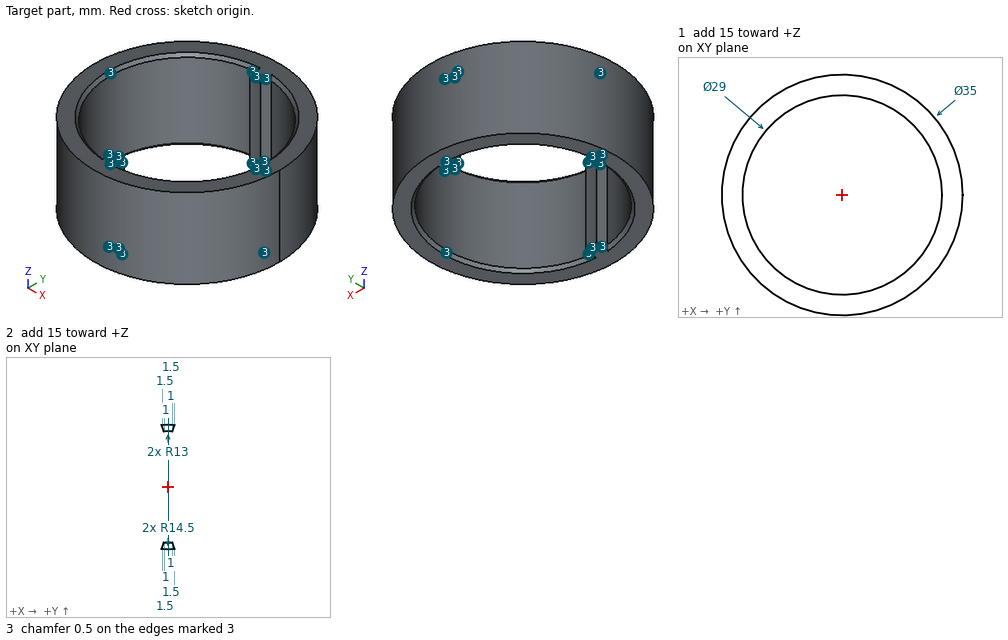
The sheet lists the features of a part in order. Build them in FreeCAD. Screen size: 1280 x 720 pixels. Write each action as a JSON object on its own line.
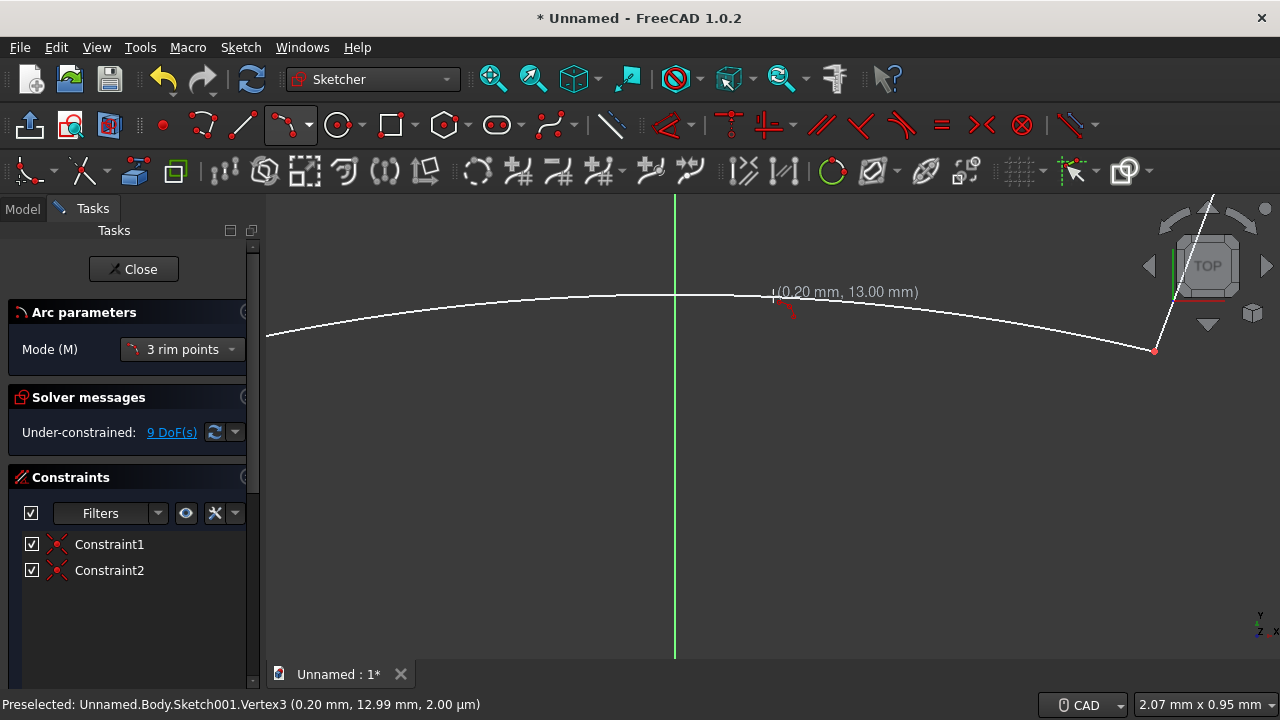
{"action": "scroll", "coordinate": [704, 426], "scroll_direction": "down", "scroll_amount": 15}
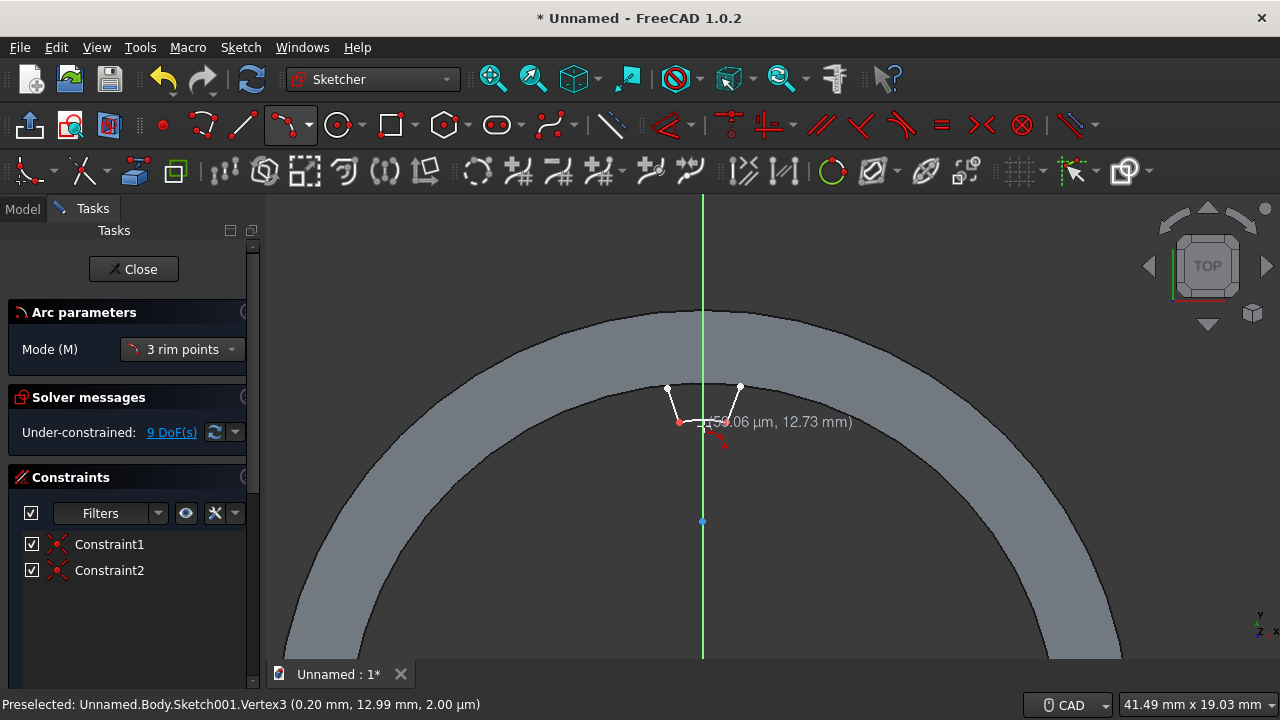
{"action": "scroll", "coordinate": [705, 245], "scroll_direction": "down", "scroll_amount": 5}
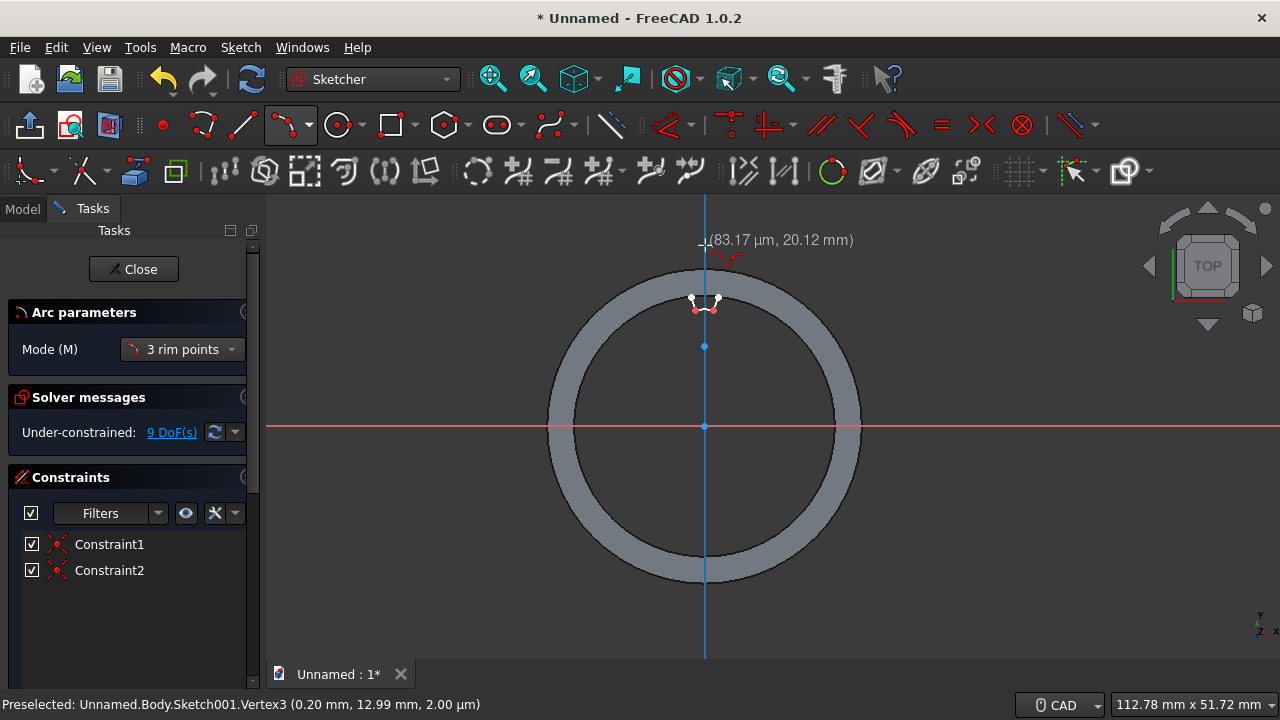
{"action": "scroll", "coordinate": [718, 297], "scroll_direction": "up", "scroll_amount": 5}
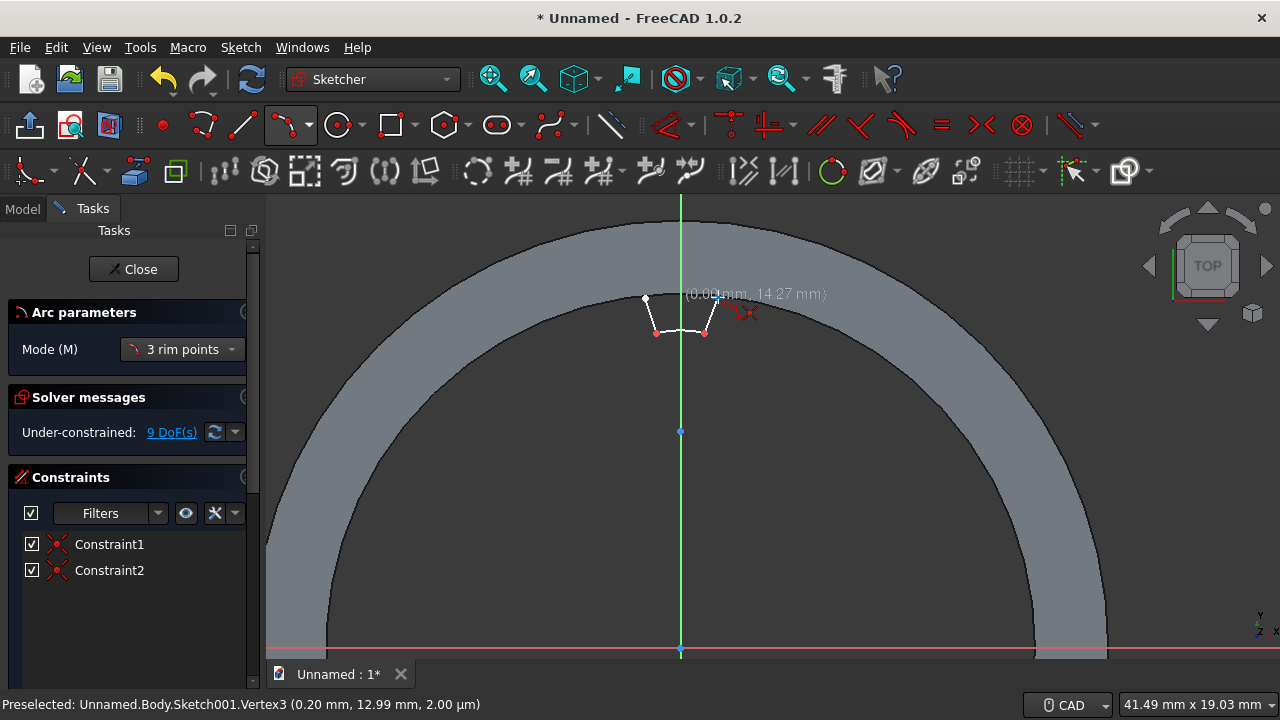
{"action": "left_click", "coordinate": [718, 297]}
{"action": "left_click", "coordinate": [645, 299]}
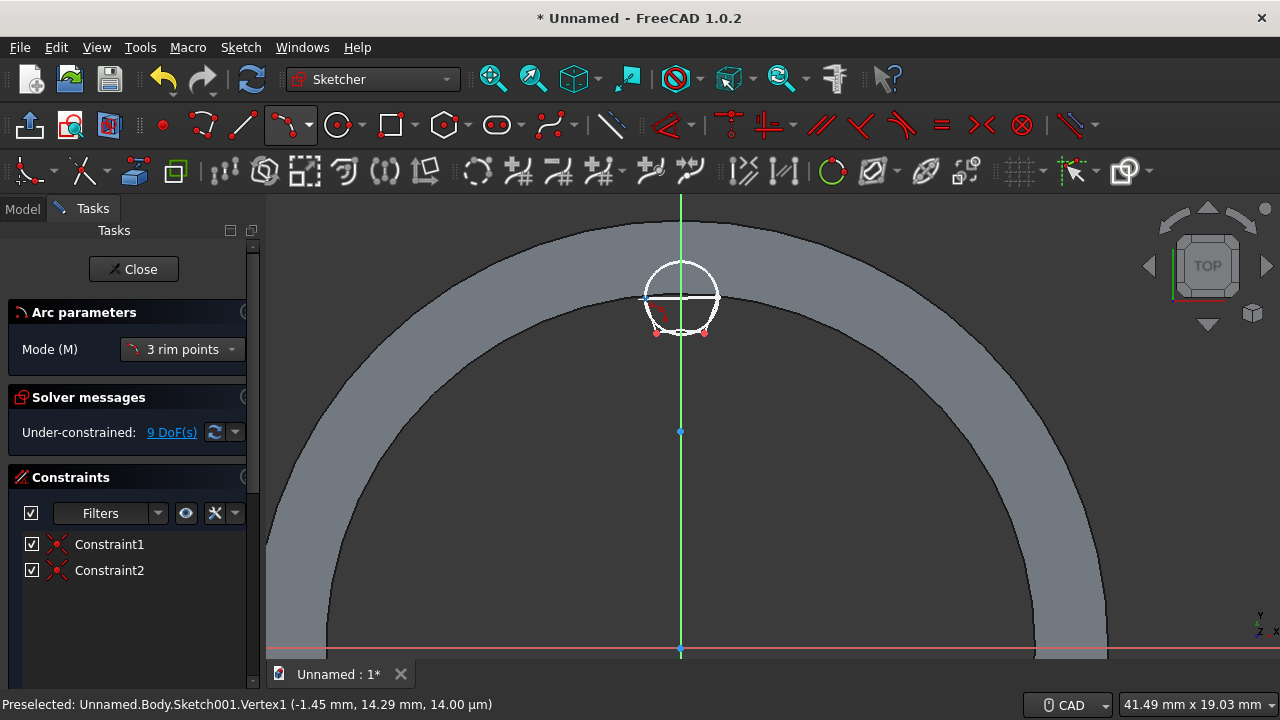
{"action": "scroll", "coordinate": [688, 294], "scroll_direction": "up", "scroll_amount": 11}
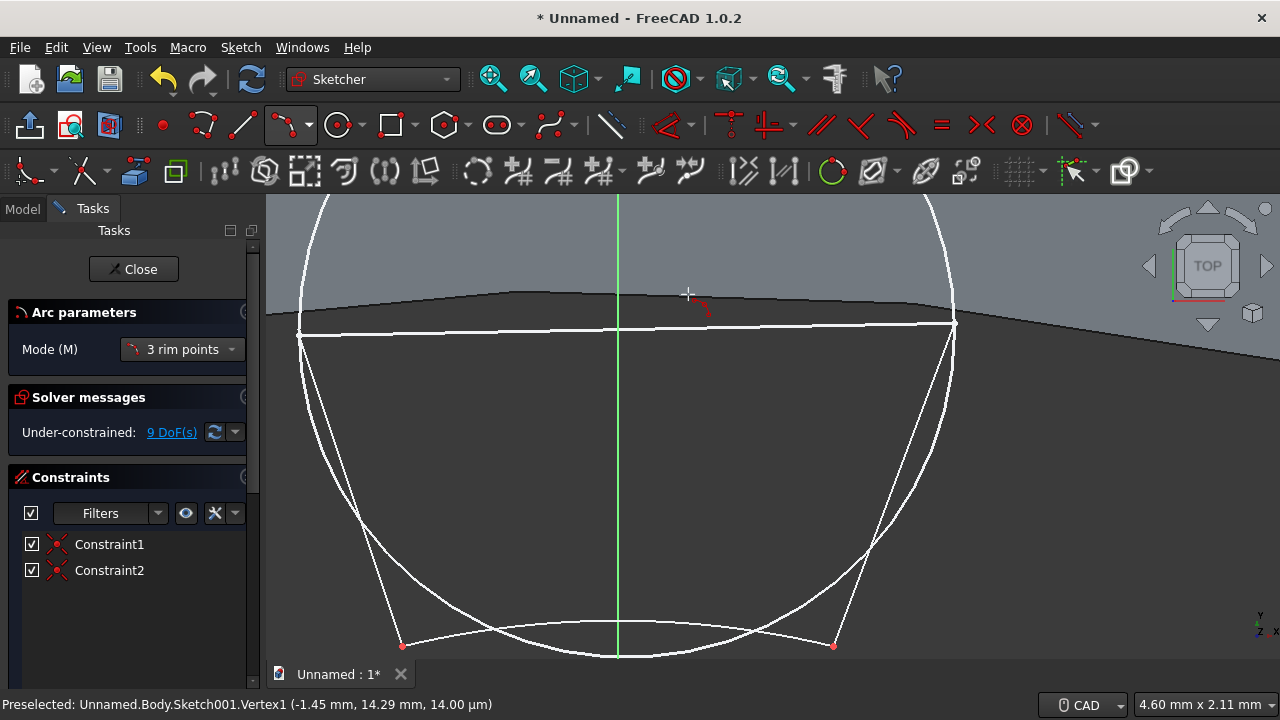
{"action": "left_click", "coordinate": [684, 291]}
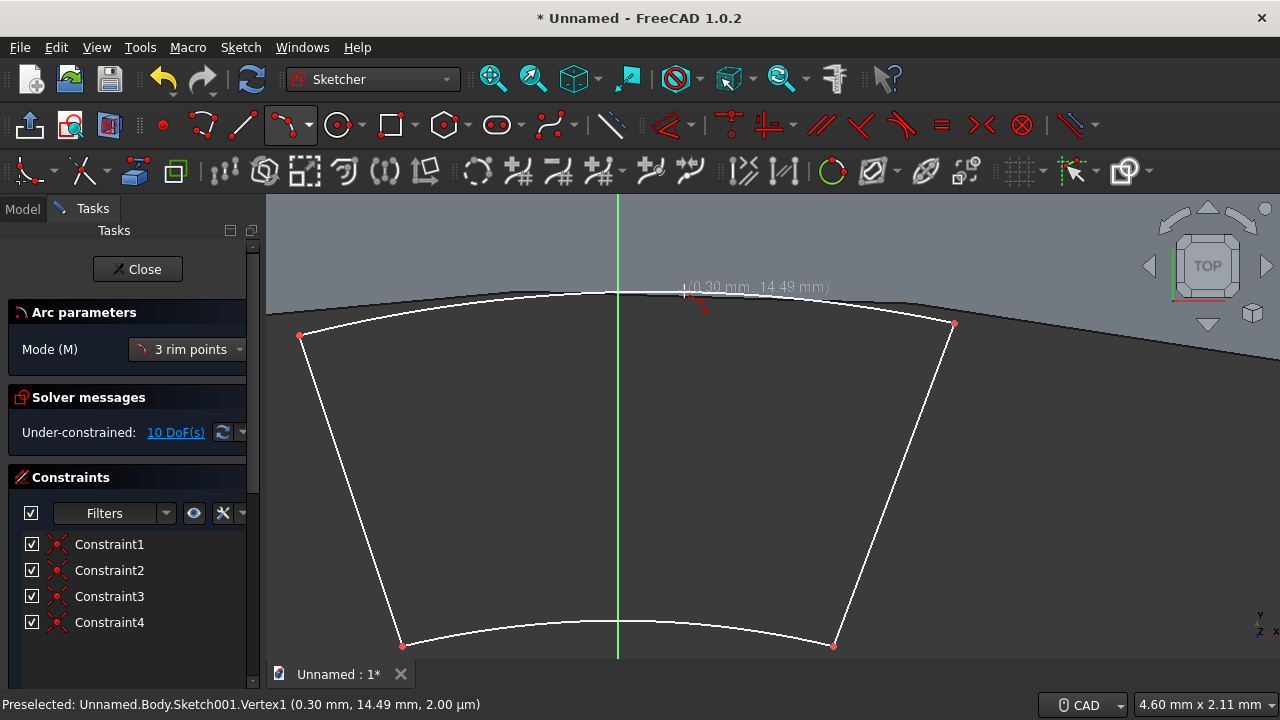
{"action": "left_click", "coordinate": [244, 126]}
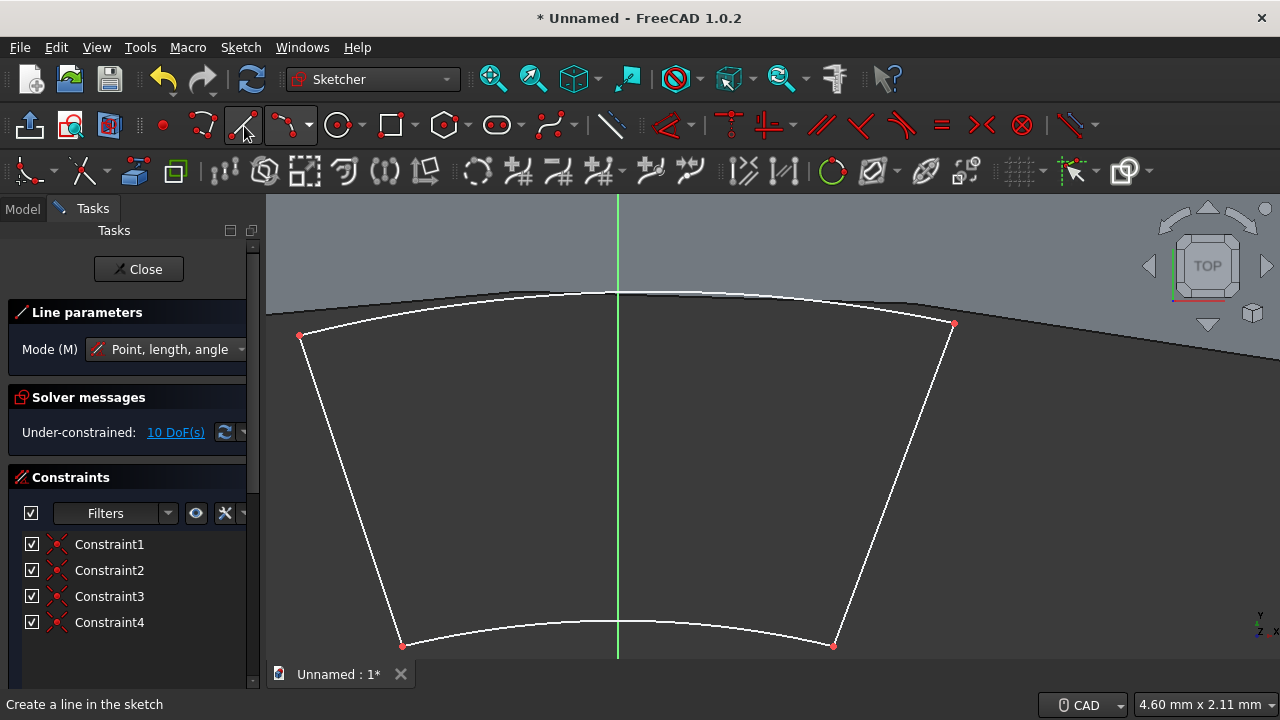
{"action": "scroll", "coordinate": [709, 266], "scroll_direction": "down", "scroll_amount": 15}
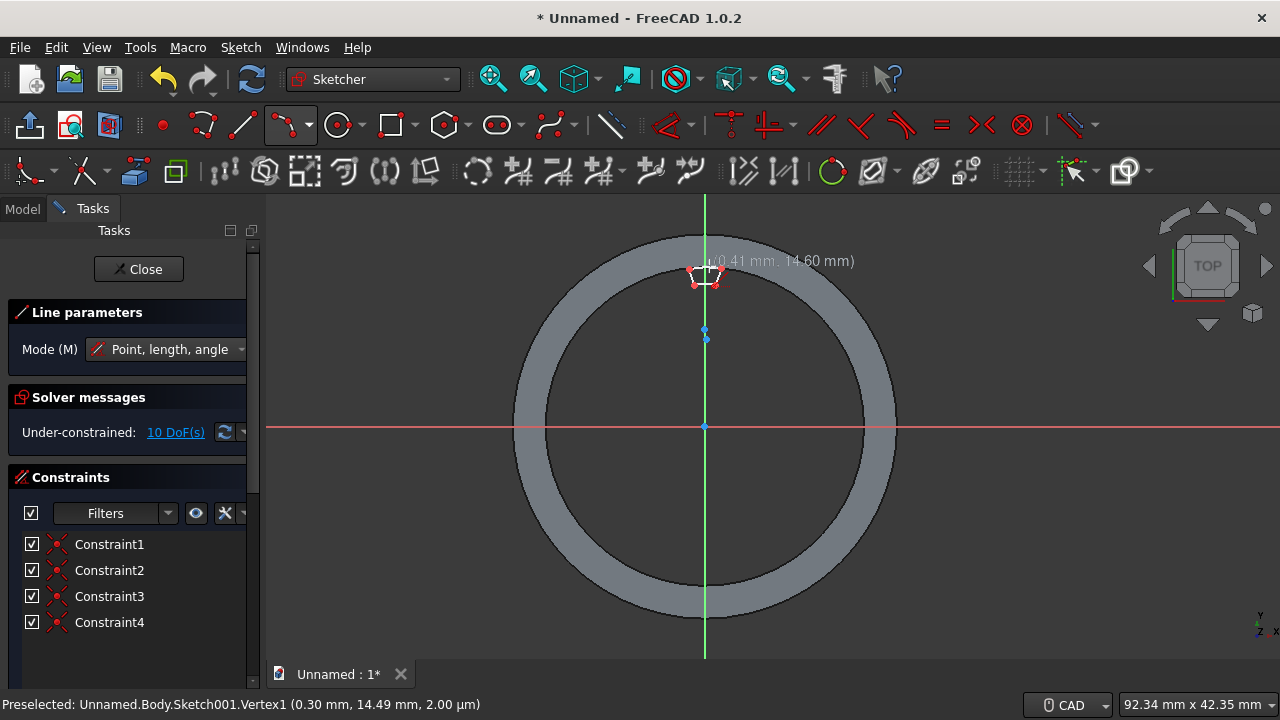
{"action": "left_click", "coordinate": [721, 585]}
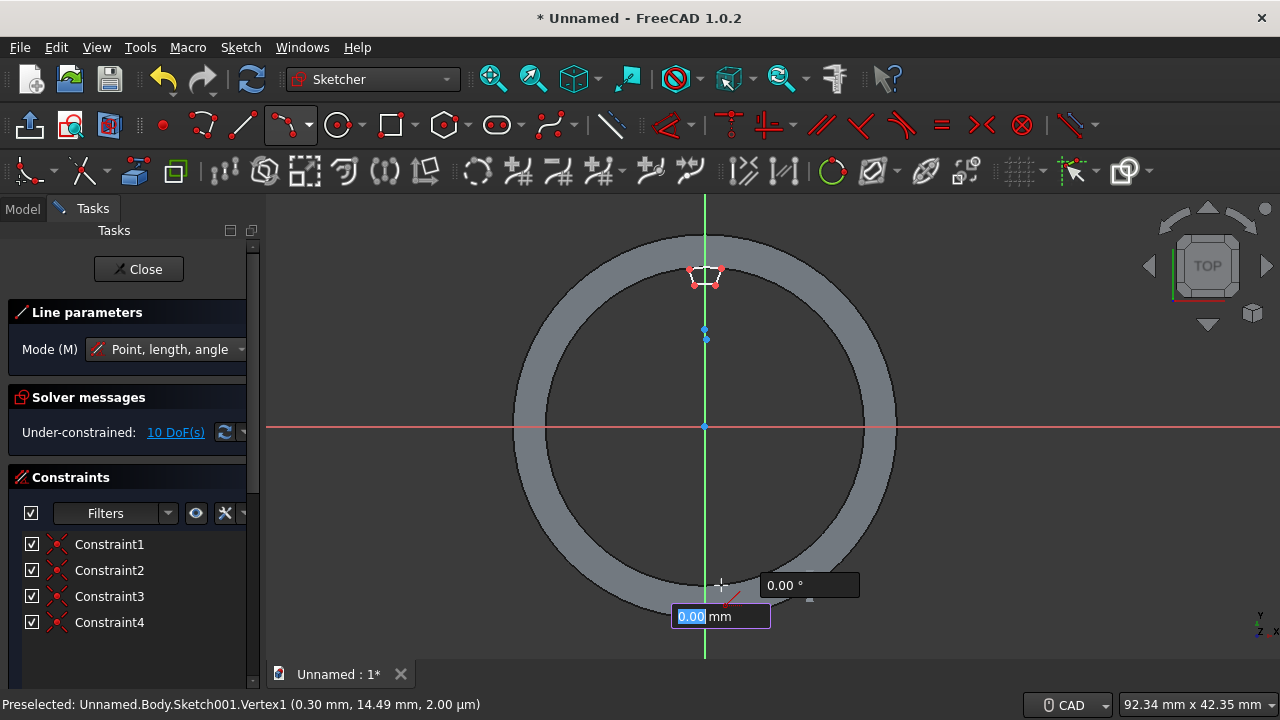
{"action": "scroll", "coordinate": [716, 569], "scroll_direction": "up", "scroll_amount": 2}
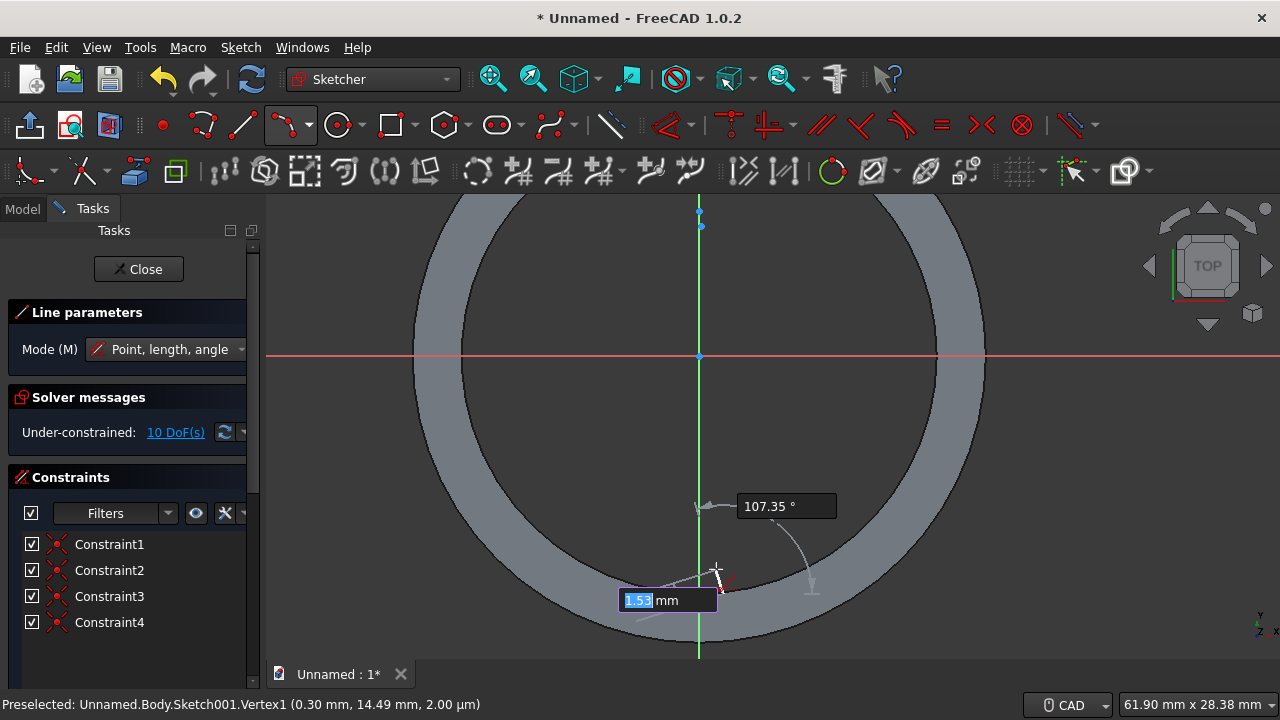
{"action": "left_click", "coordinate": [716, 568]}